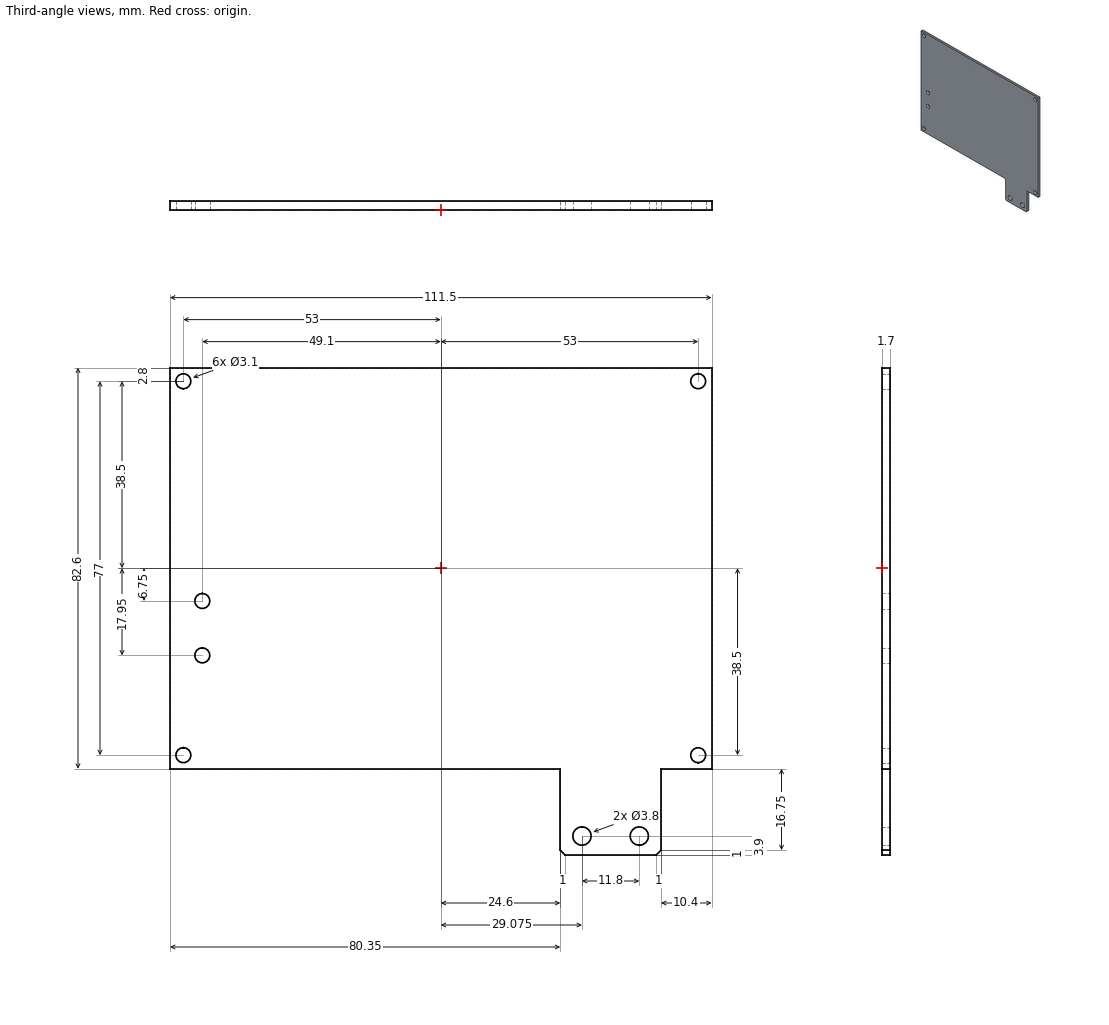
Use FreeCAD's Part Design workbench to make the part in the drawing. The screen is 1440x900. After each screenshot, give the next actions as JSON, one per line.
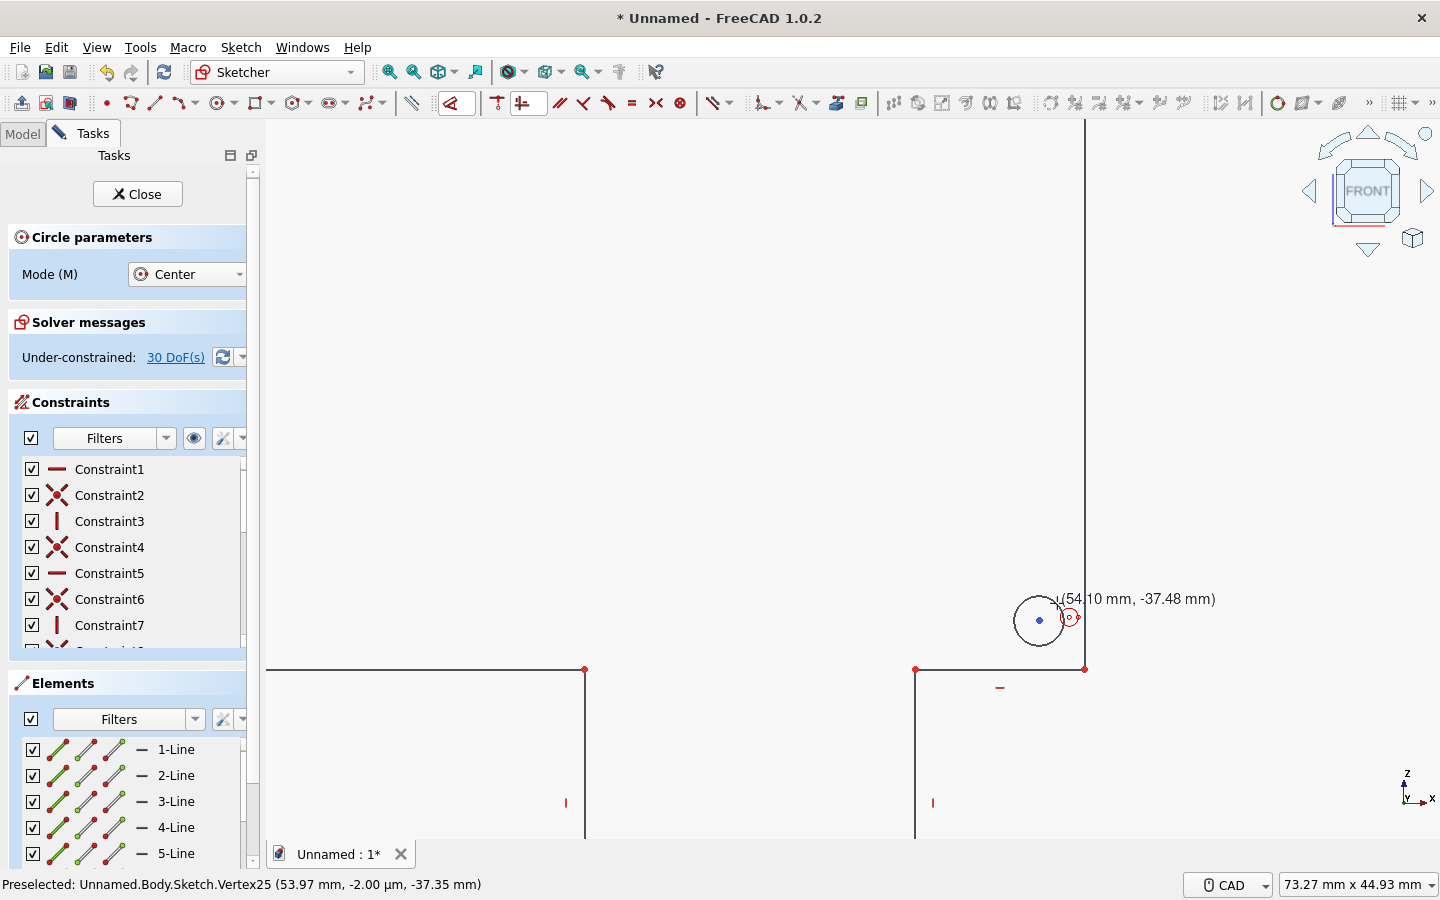
{"action": "scroll", "coordinate": [1041, 623], "scroll_direction": "down", "scroll_amount": 6}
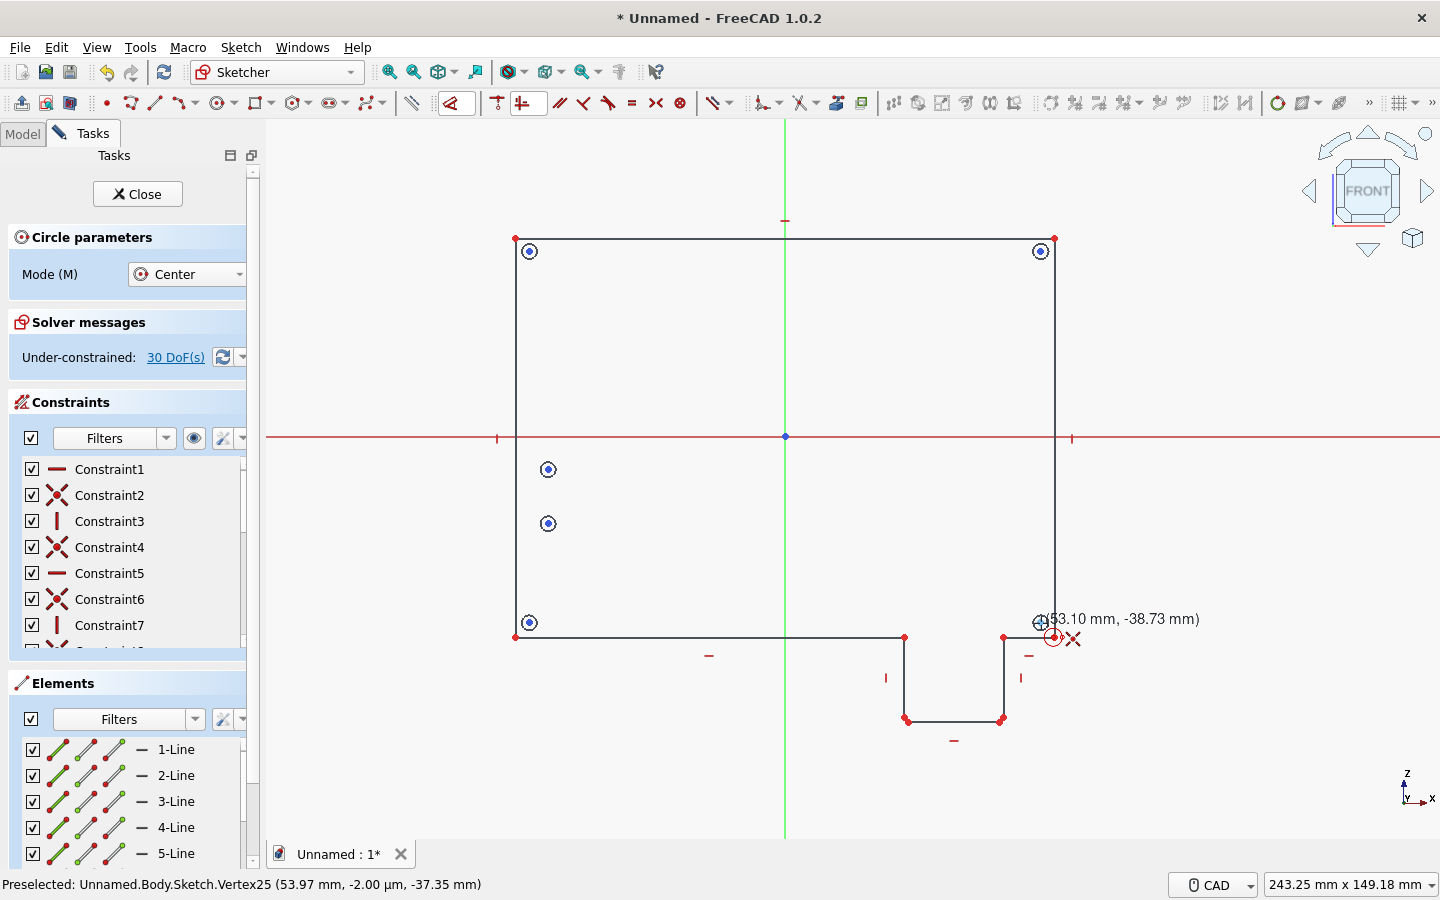
{"action": "scroll", "coordinate": [925, 703], "scroll_direction": "up", "scroll_amount": 5}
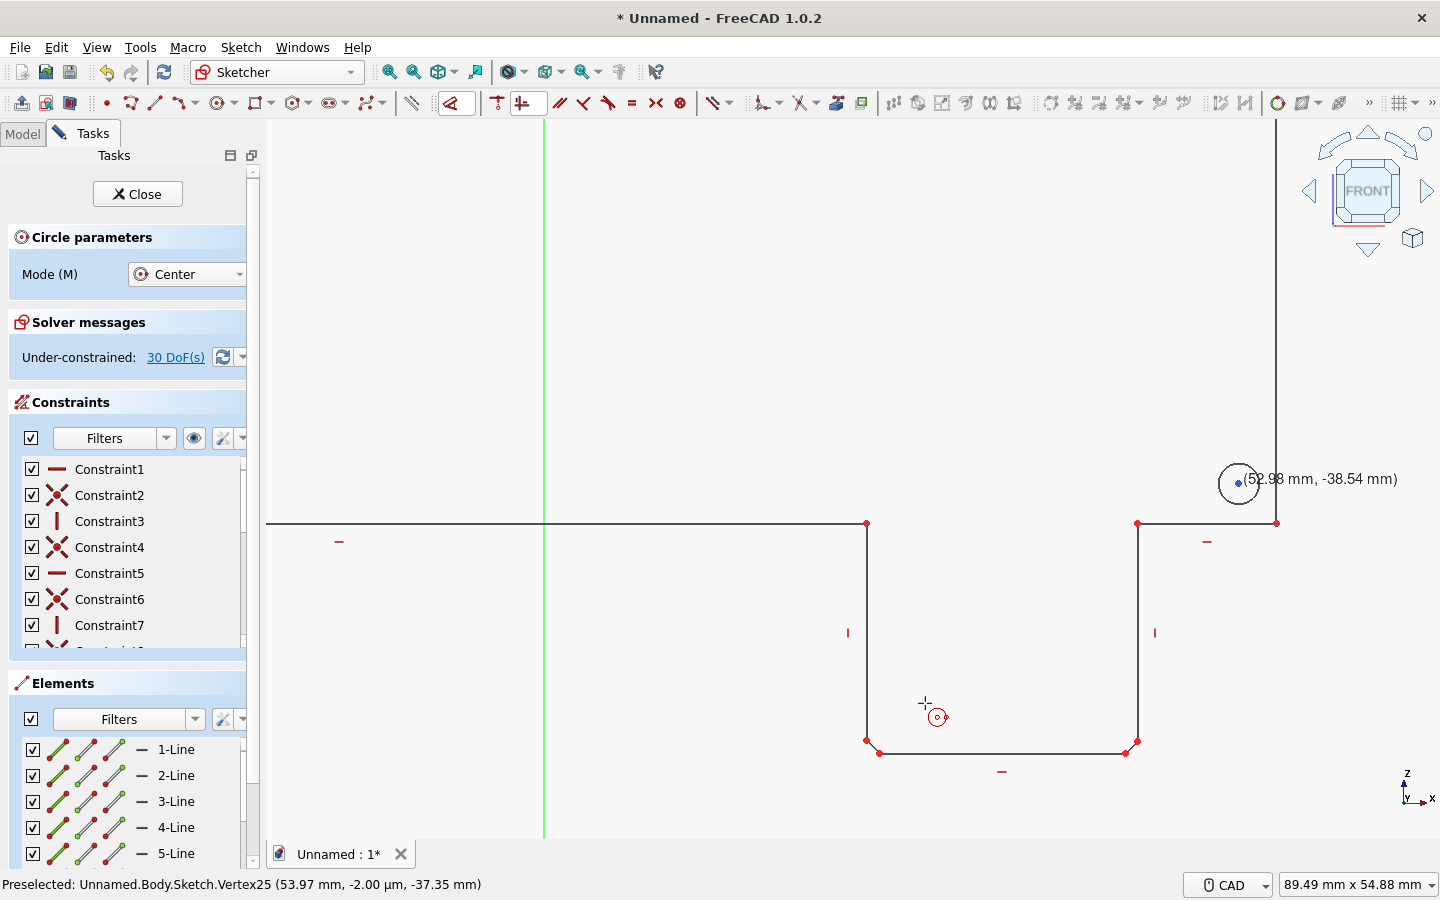
{"action": "left_click", "coordinate": [925, 702]}
{"action": "left_click", "coordinate": [943, 684]}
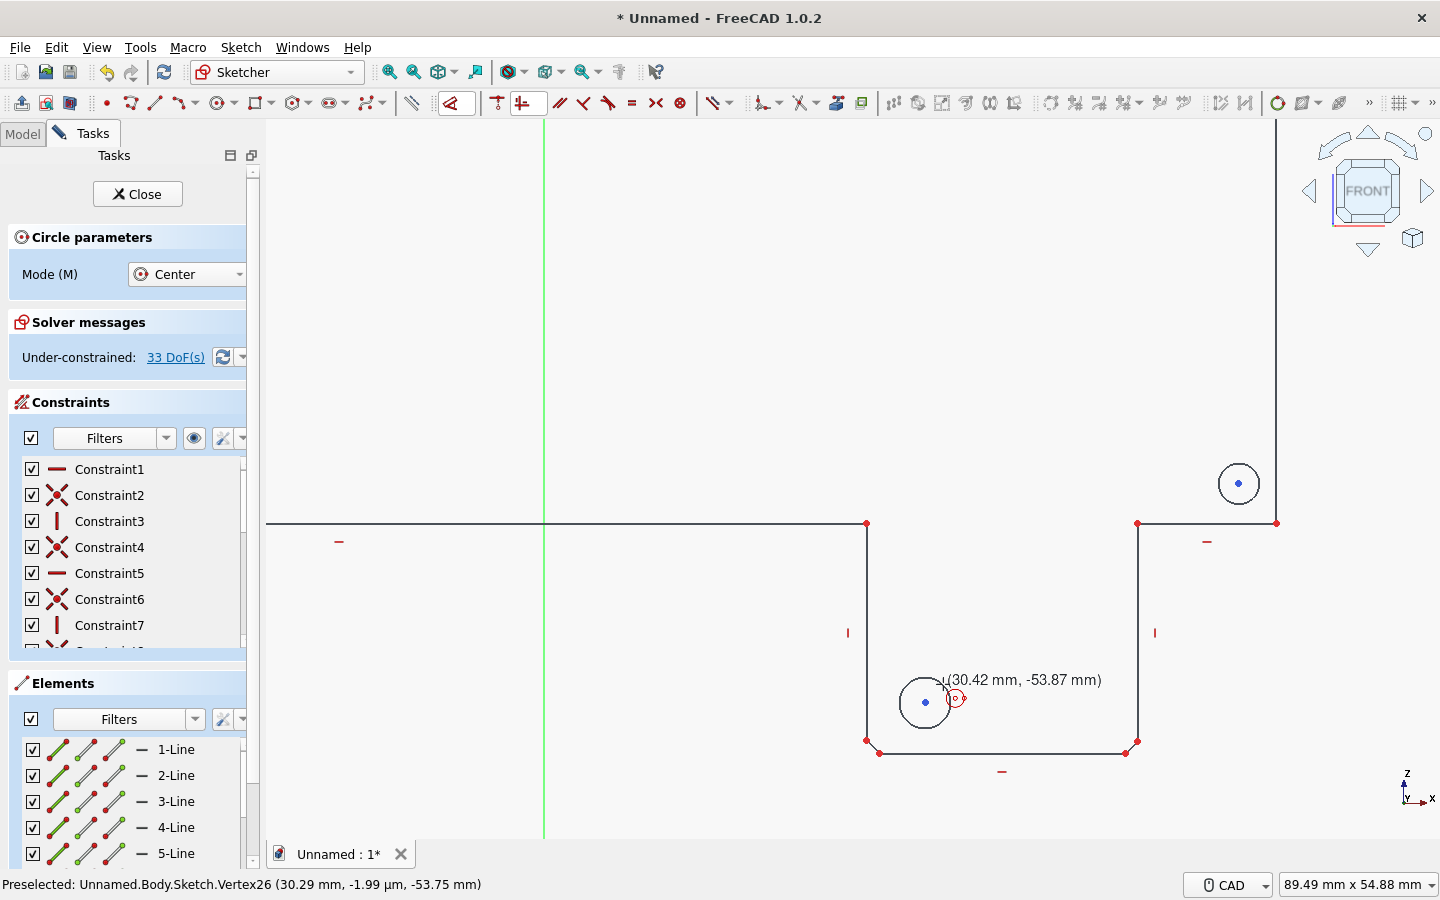
{"action": "left_click", "coordinate": [1080, 702]}
{"action": "left_click", "coordinate": [1098, 684]}
{"action": "key", "text": "Escape"}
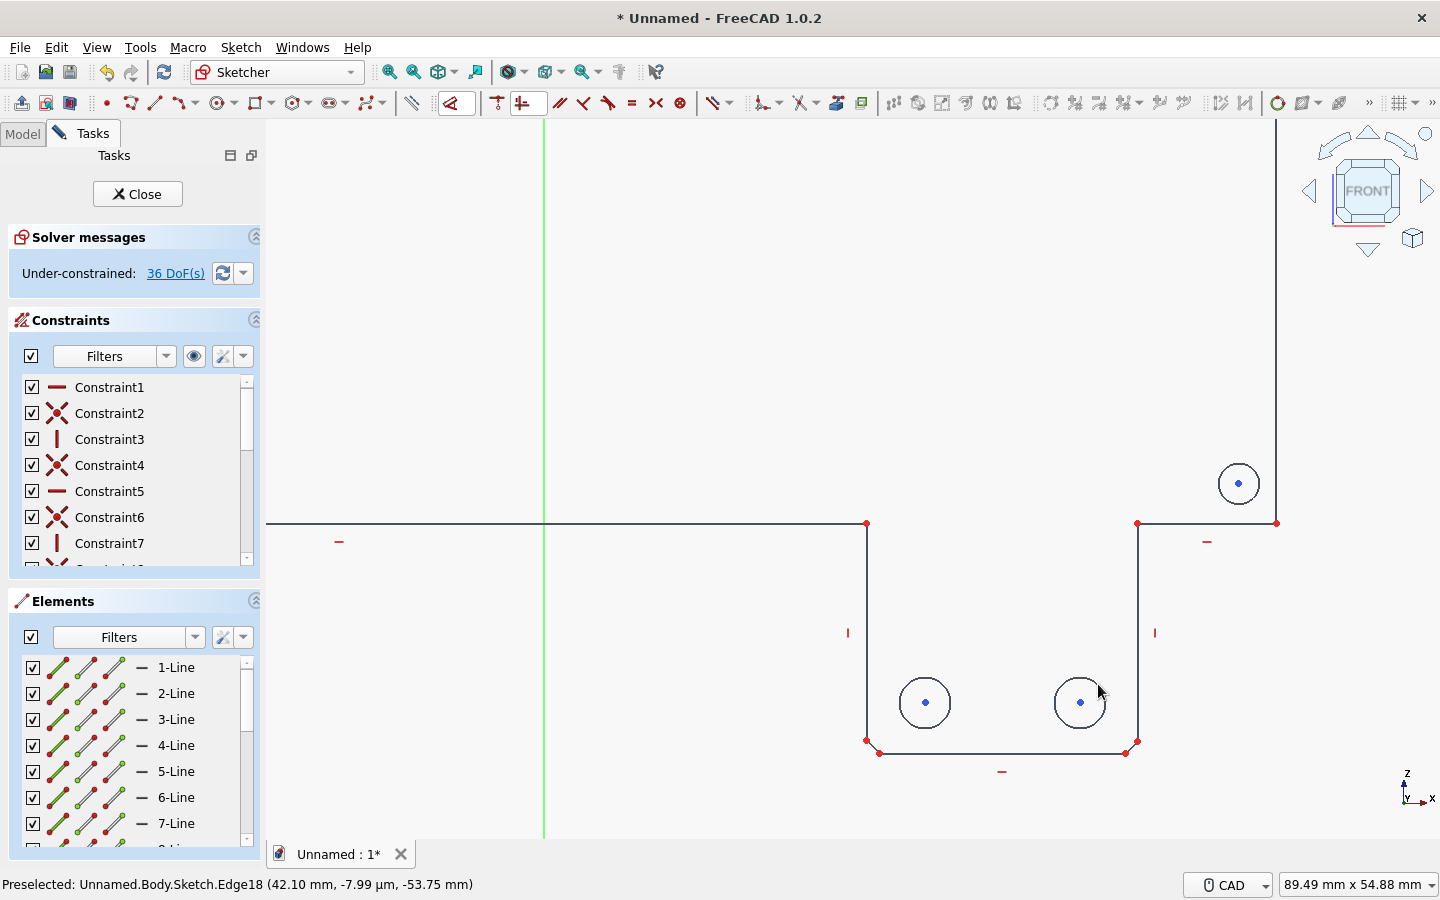
{"action": "scroll", "coordinate": [925, 703], "scroll_direction": "down", "scroll_amount": 5}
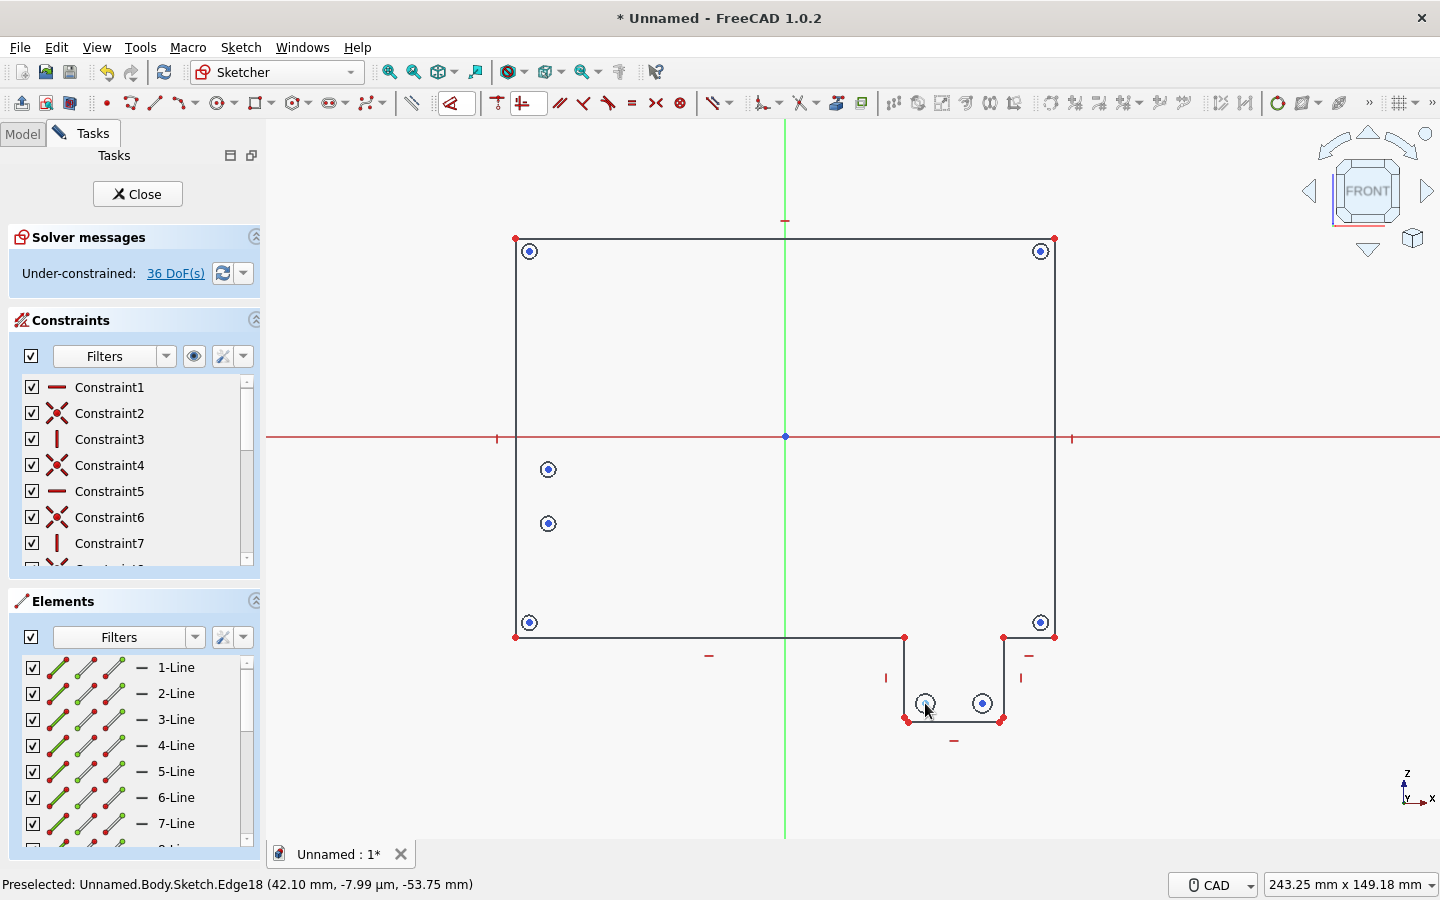
{"action": "scroll", "coordinate": [535, 246], "scroll_direction": "up", "scroll_amount": 4}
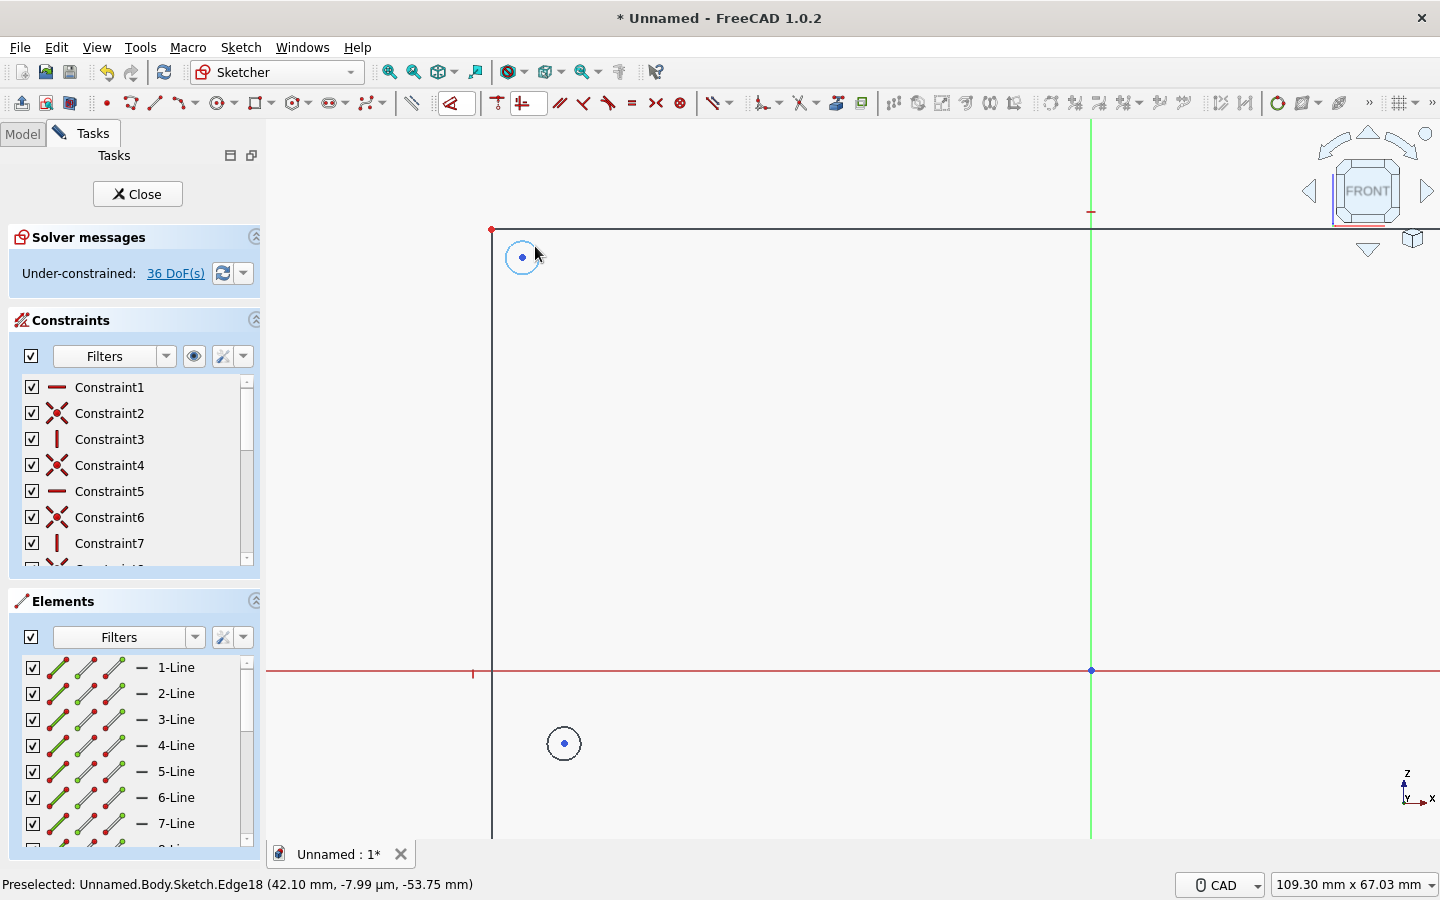
{"action": "left_click", "coordinate": [534, 246]}